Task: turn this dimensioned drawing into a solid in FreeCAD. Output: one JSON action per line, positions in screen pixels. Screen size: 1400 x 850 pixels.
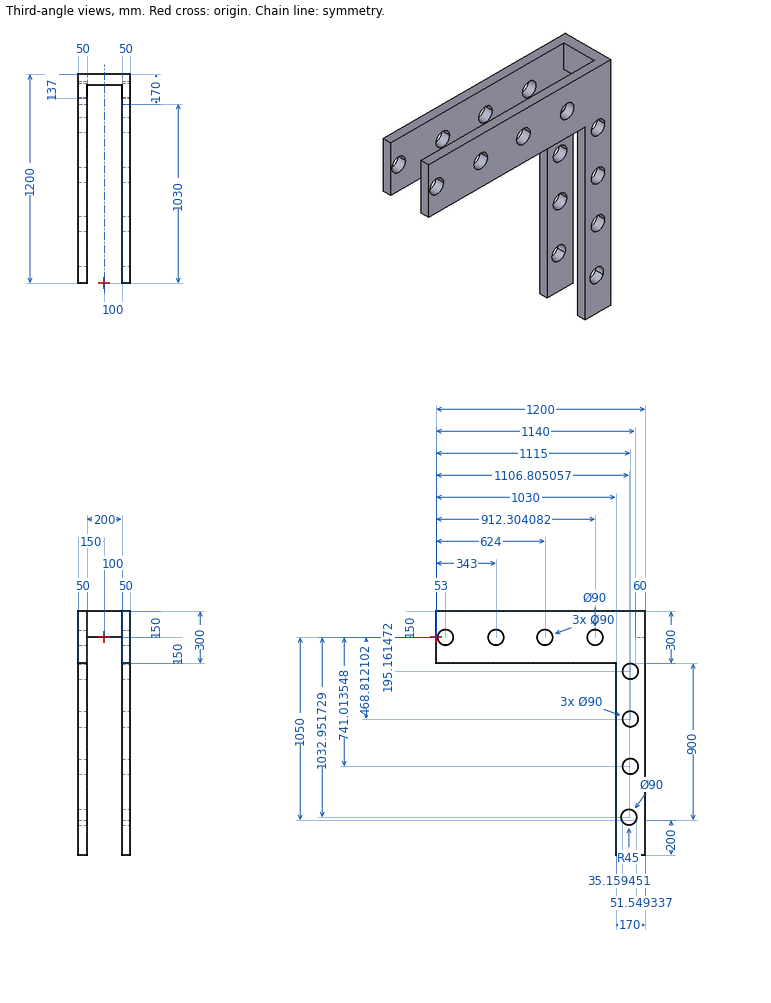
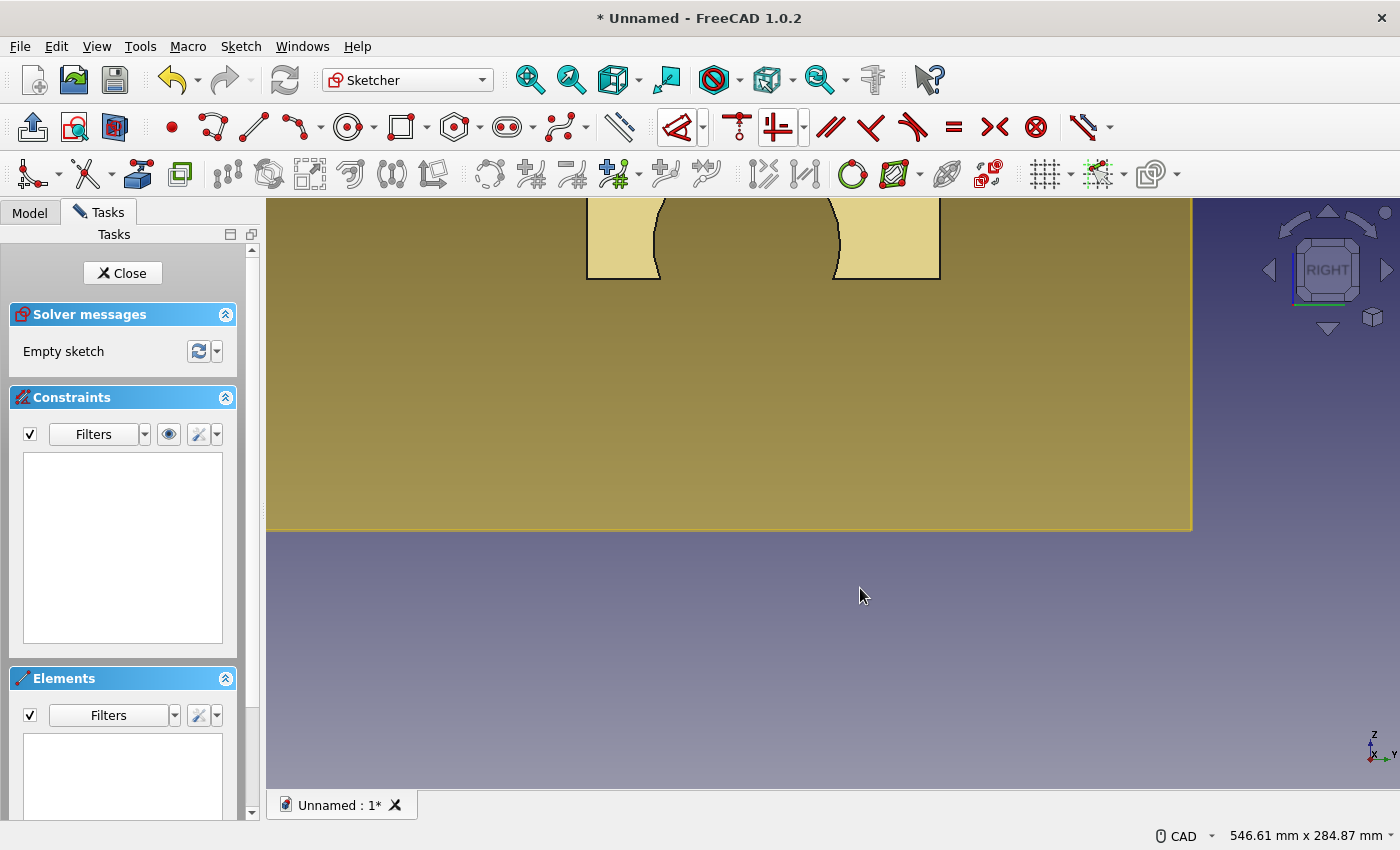
{"action": "left_click", "coordinate": [213, 128]}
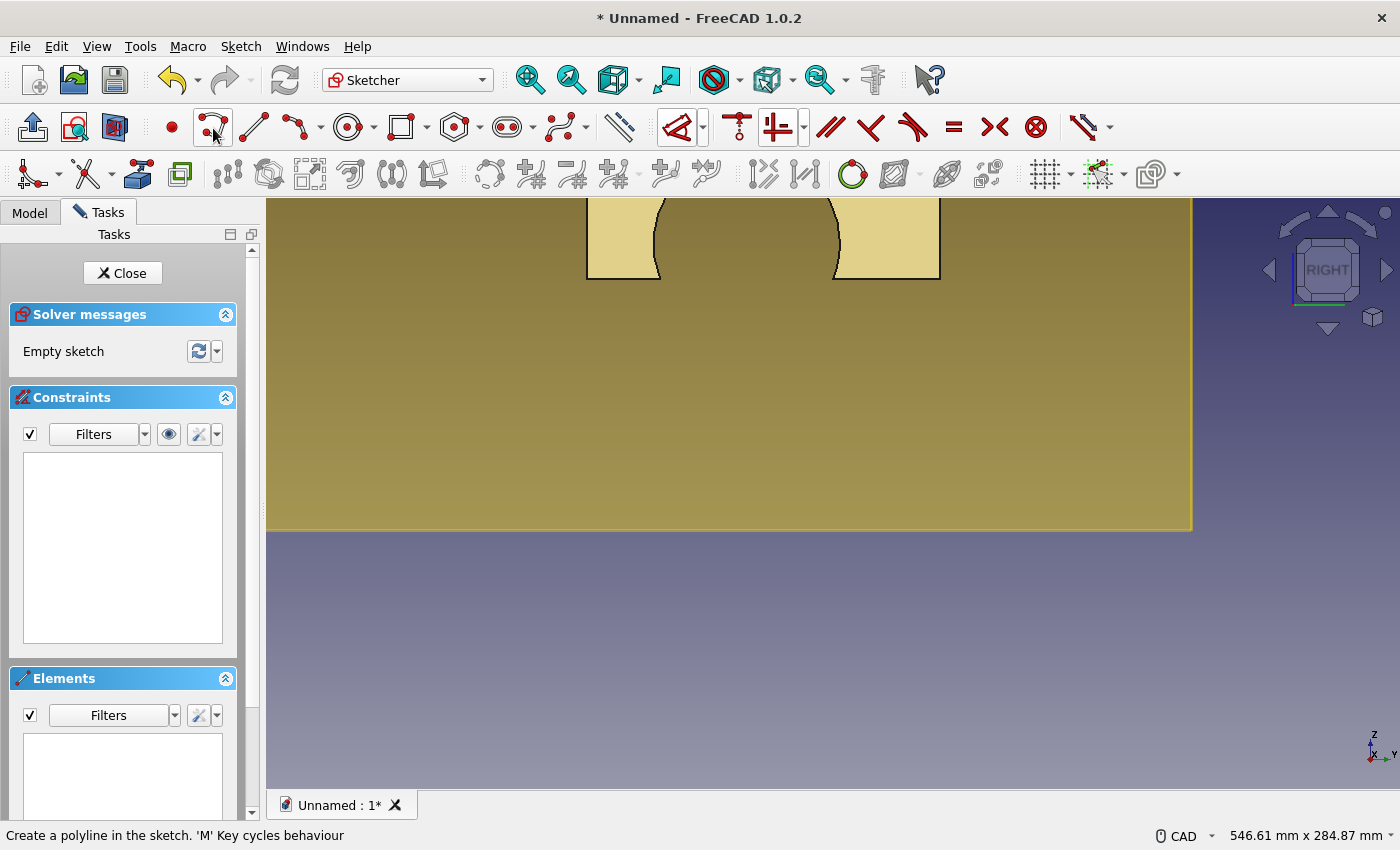
{"action": "left_click", "coordinate": [833, 279]}
{"action": "left_click", "coordinate": [940, 279]}
{"action": "left_click", "coordinate": [940, 694]}
{"action": "left_click", "coordinate": [587, 694]}
{"action": "left_click", "coordinate": [587, 279]}
{"action": "left_click", "coordinate": [660, 279]}
{"action": "right_click", "coordinate": [660, 279]}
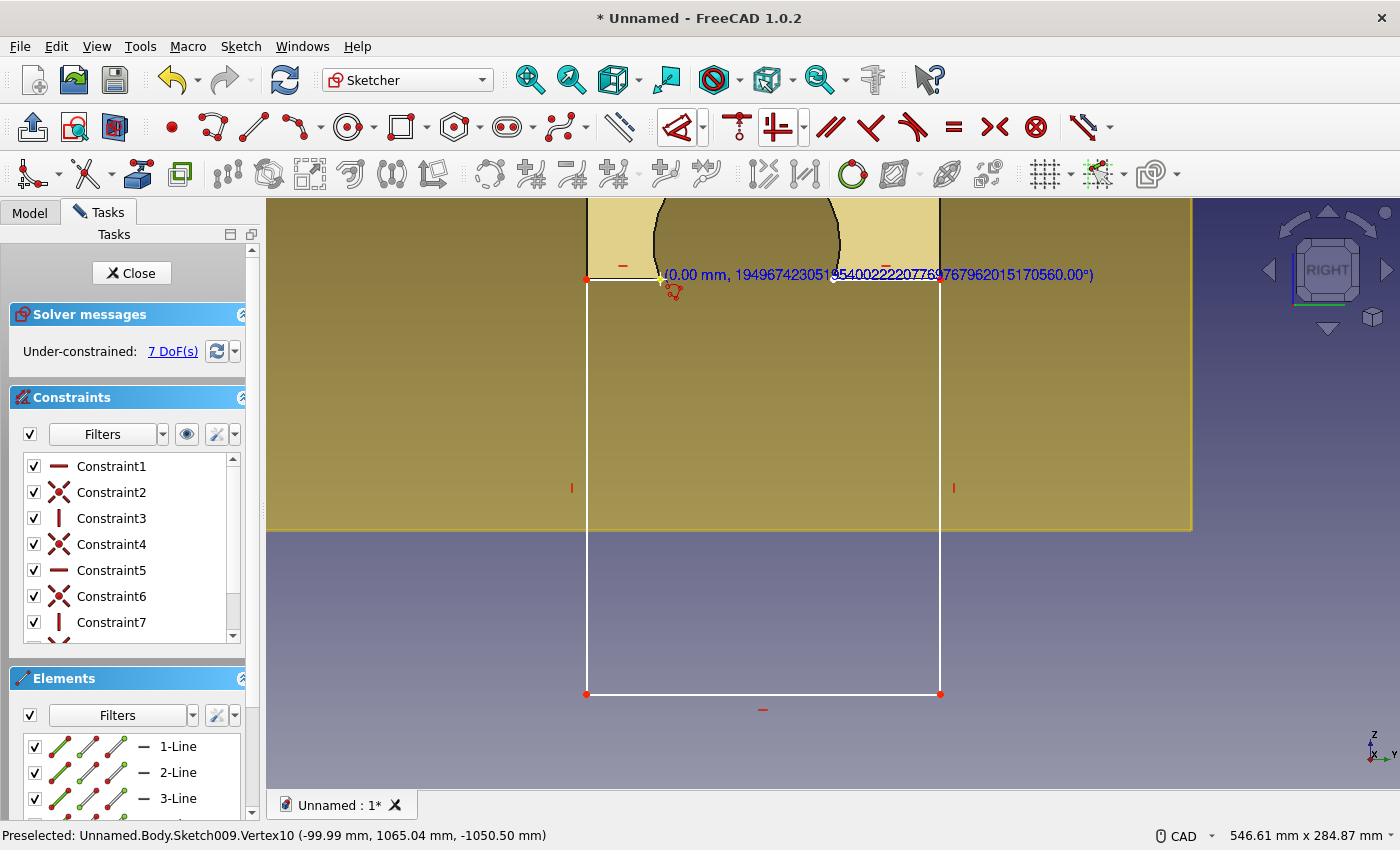
{"action": "left_click", "coordinate": [294, 128]}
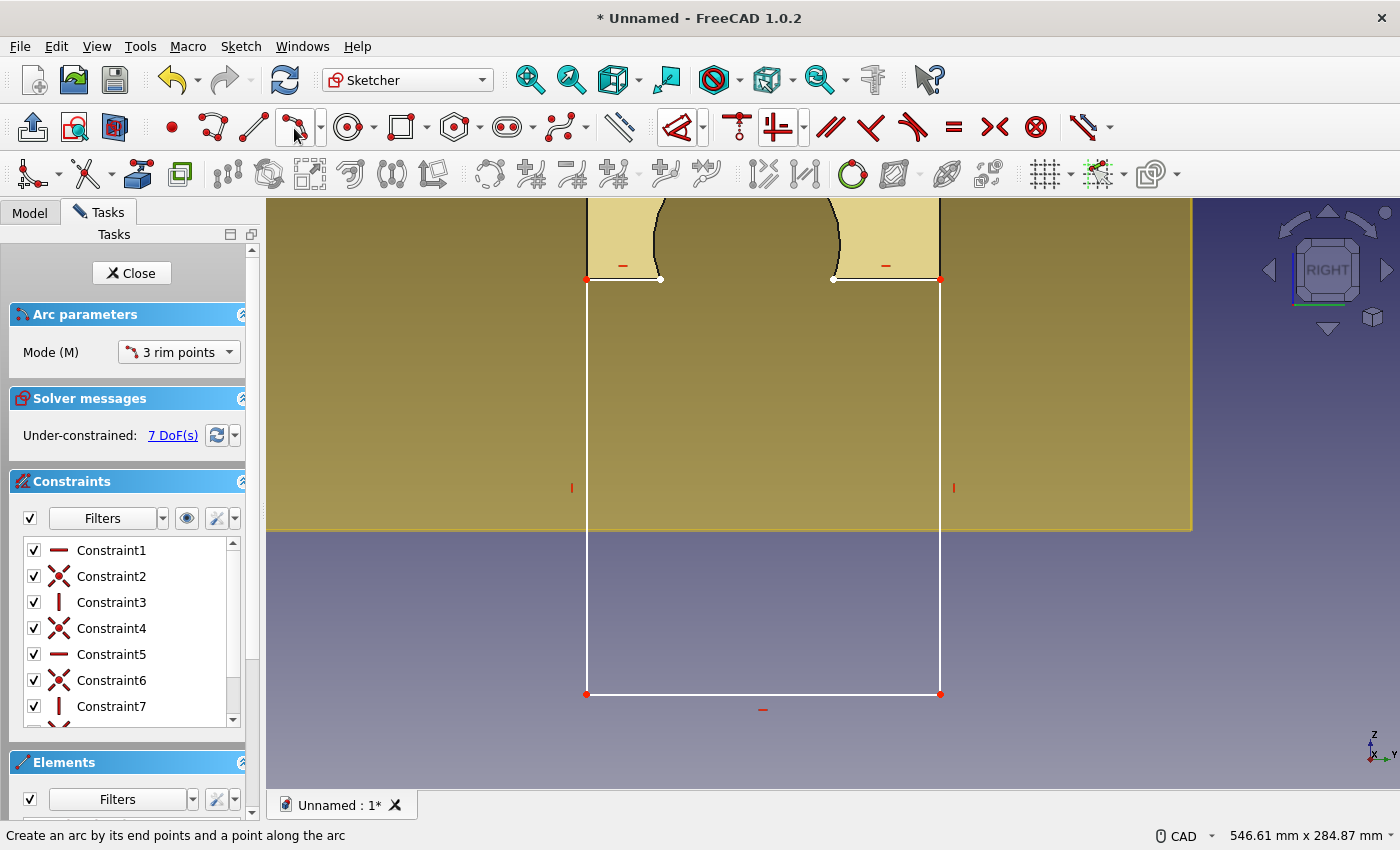
{"action": "left_click", "coordinate": [660, 280]}
{"action": "left_click", "coordinate": [833, 280]}
{"action": "left_click", "coordinate": [747, 337]}
{"action": "key", "text": "Escape"}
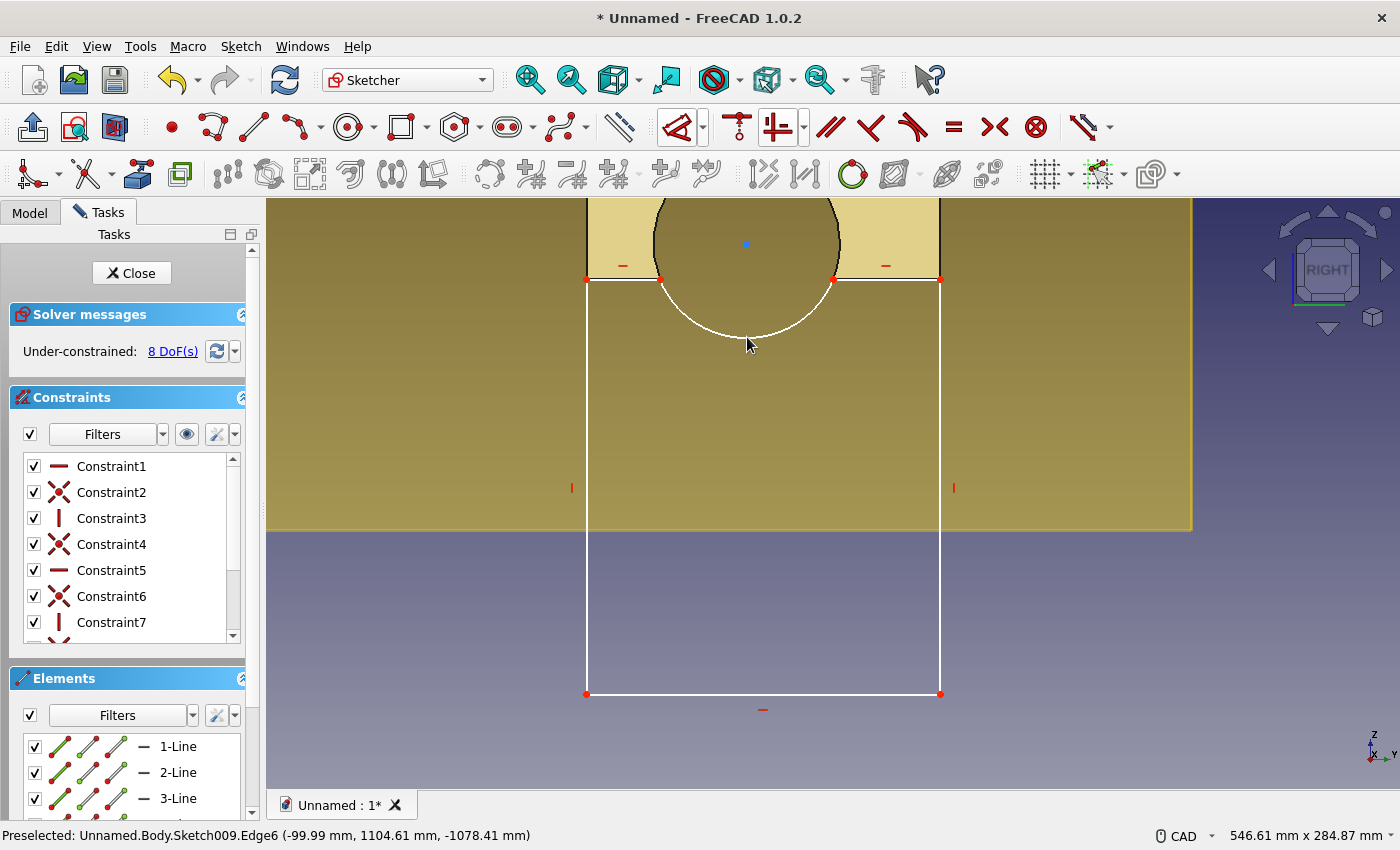
{"action": "left_click", "coordinate": [704, 328]}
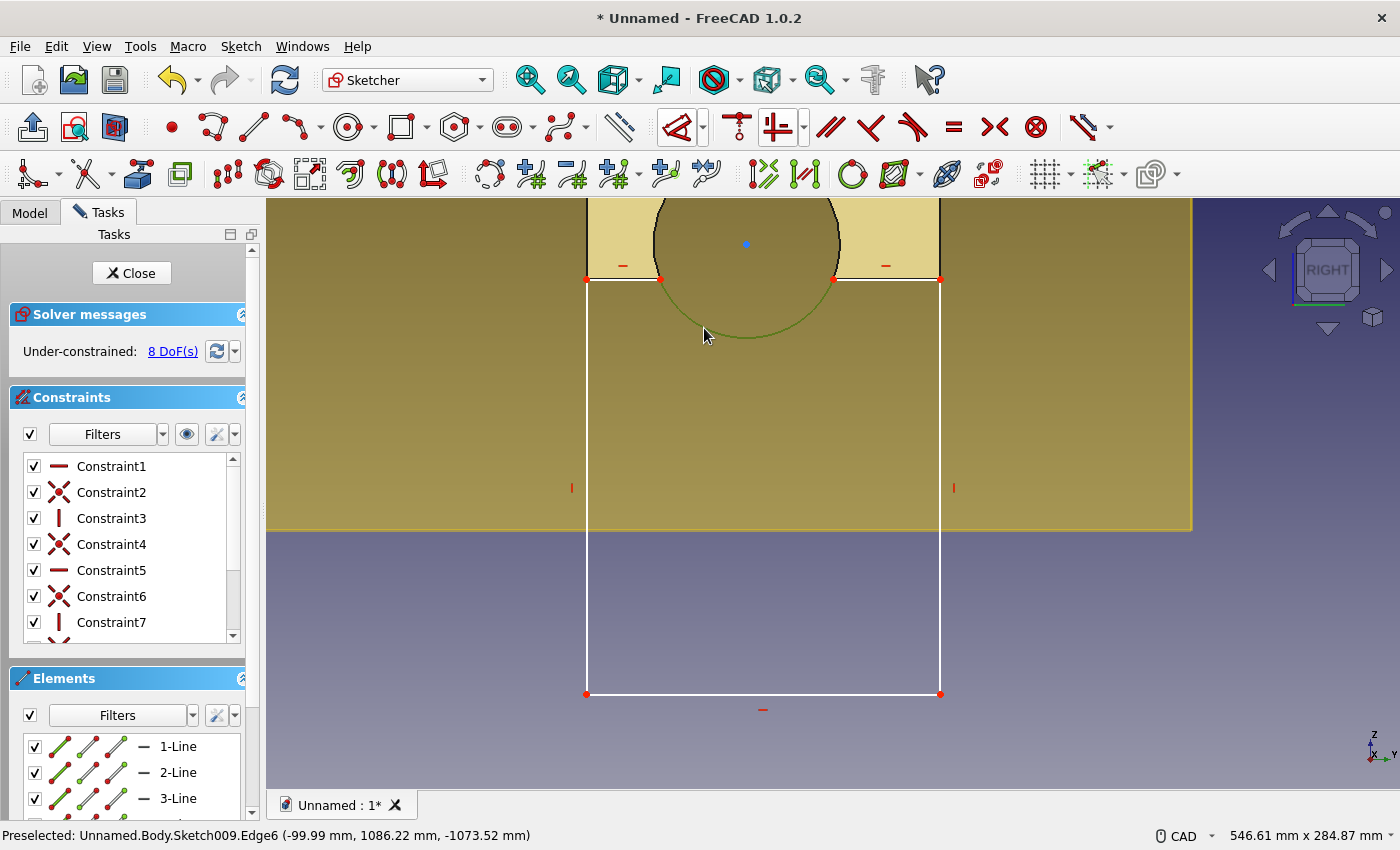
{"action": "key", "text": "k r"}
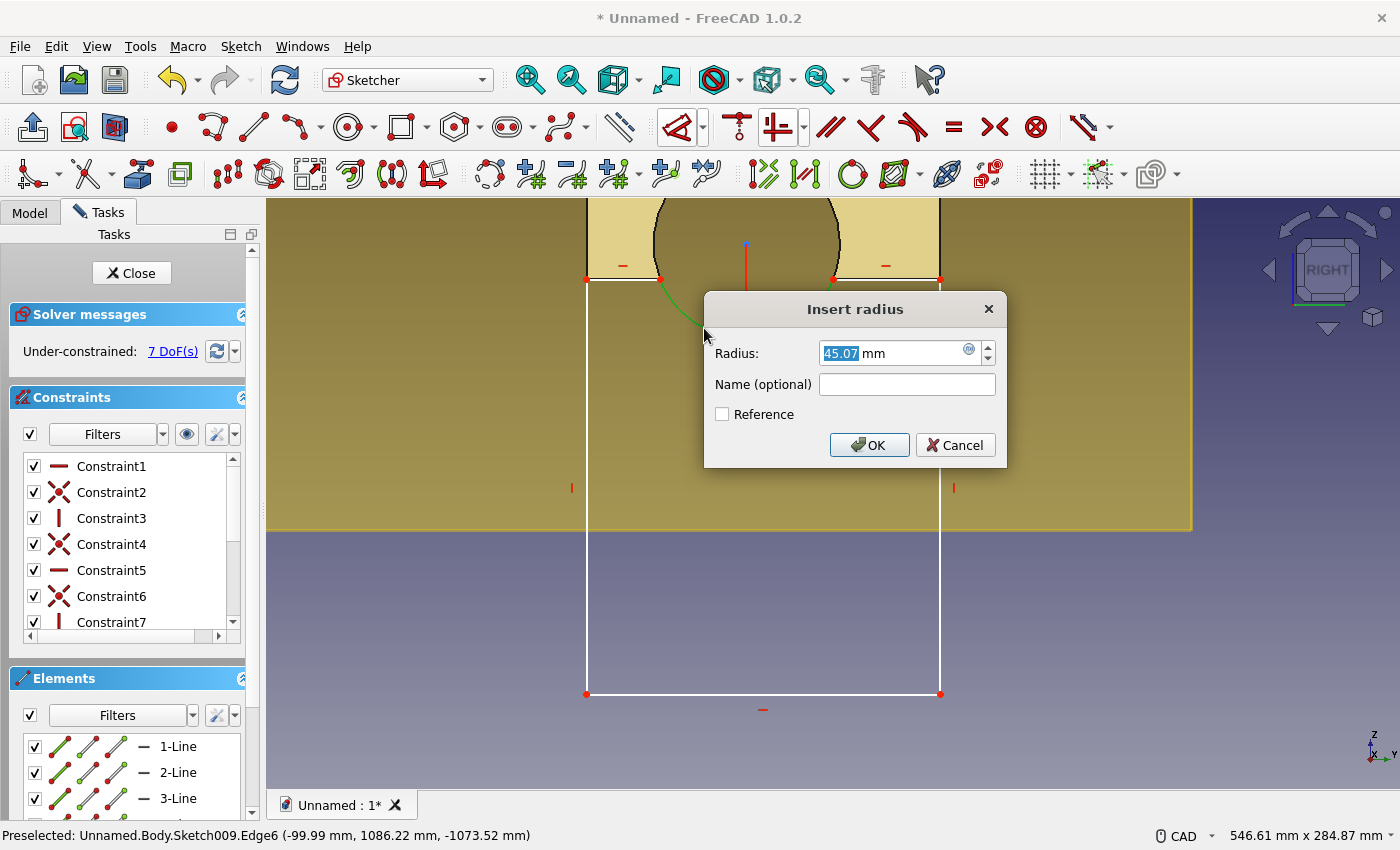
{"action": "type", "text": "45"}
{"action": "key", "text": "Return"}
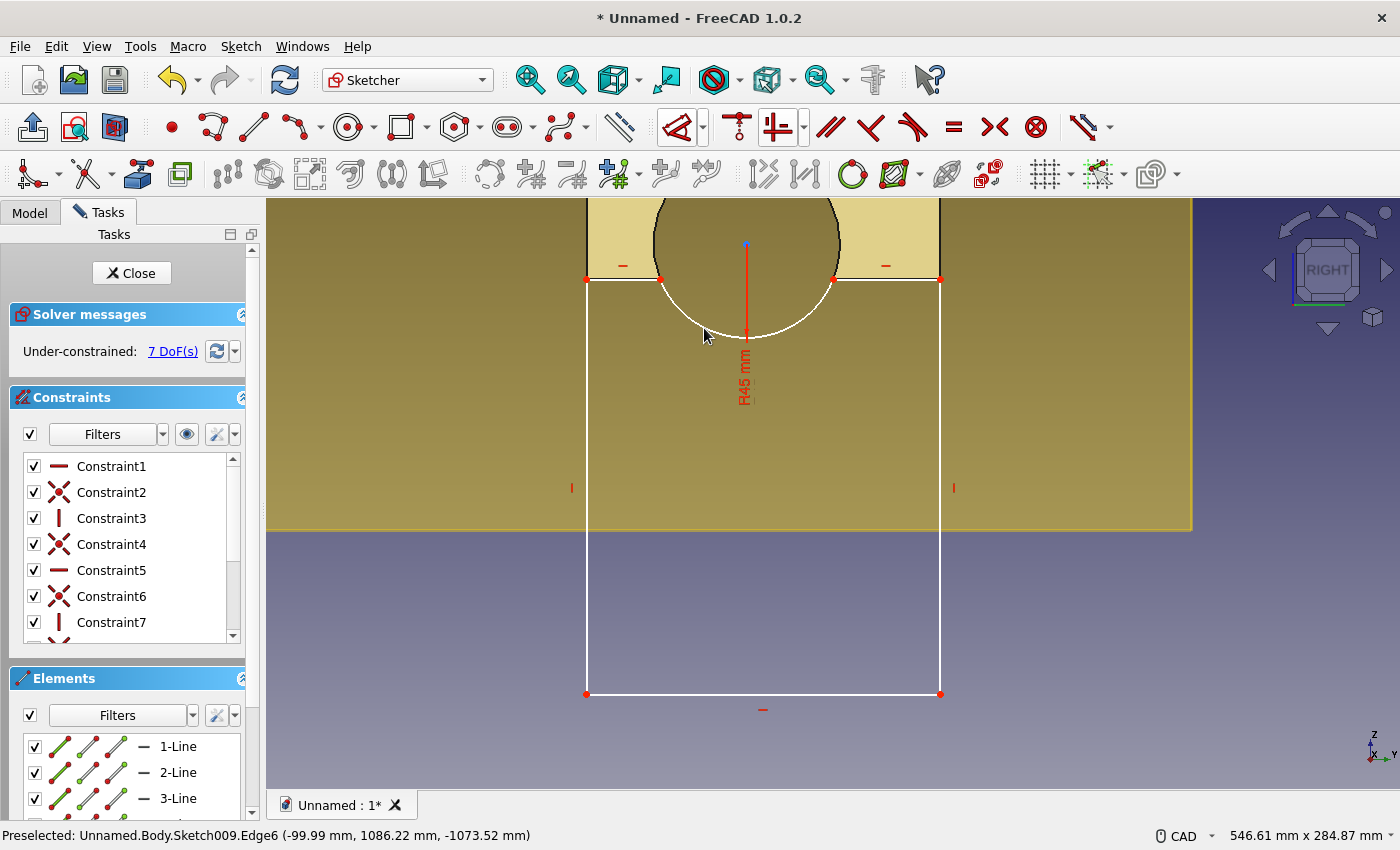
{"action": "left_click", "coordinate": [940, 405]}